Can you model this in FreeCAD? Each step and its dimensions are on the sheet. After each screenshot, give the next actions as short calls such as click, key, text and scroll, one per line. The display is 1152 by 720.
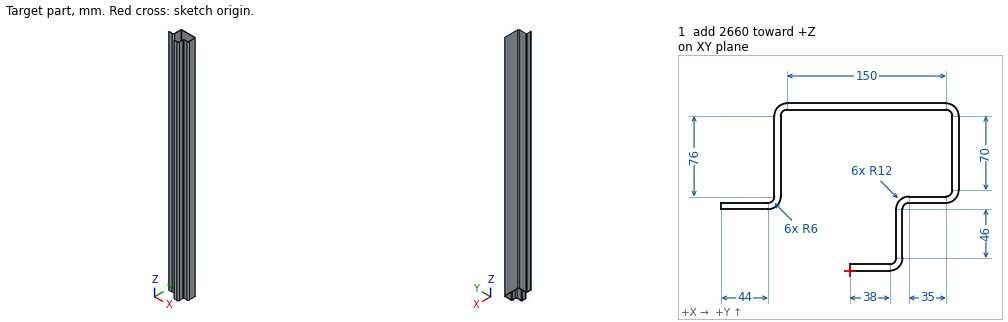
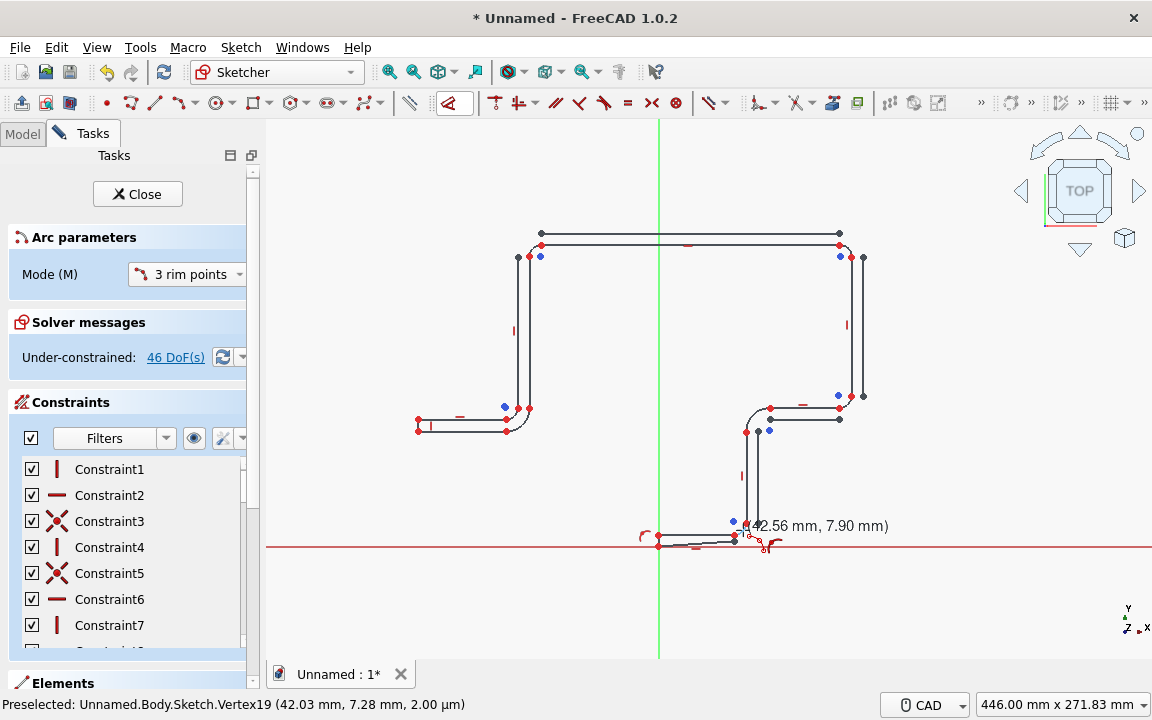
scroll(734, 547, up, 2)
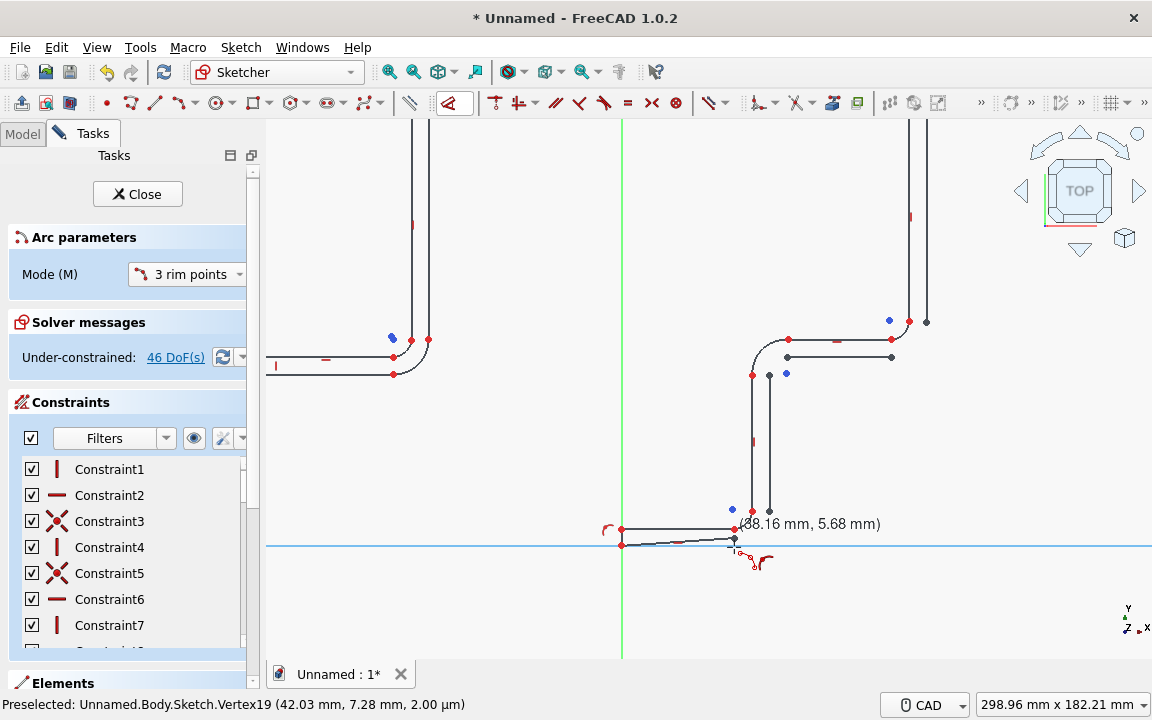
click(735, 538)
click(770, 511)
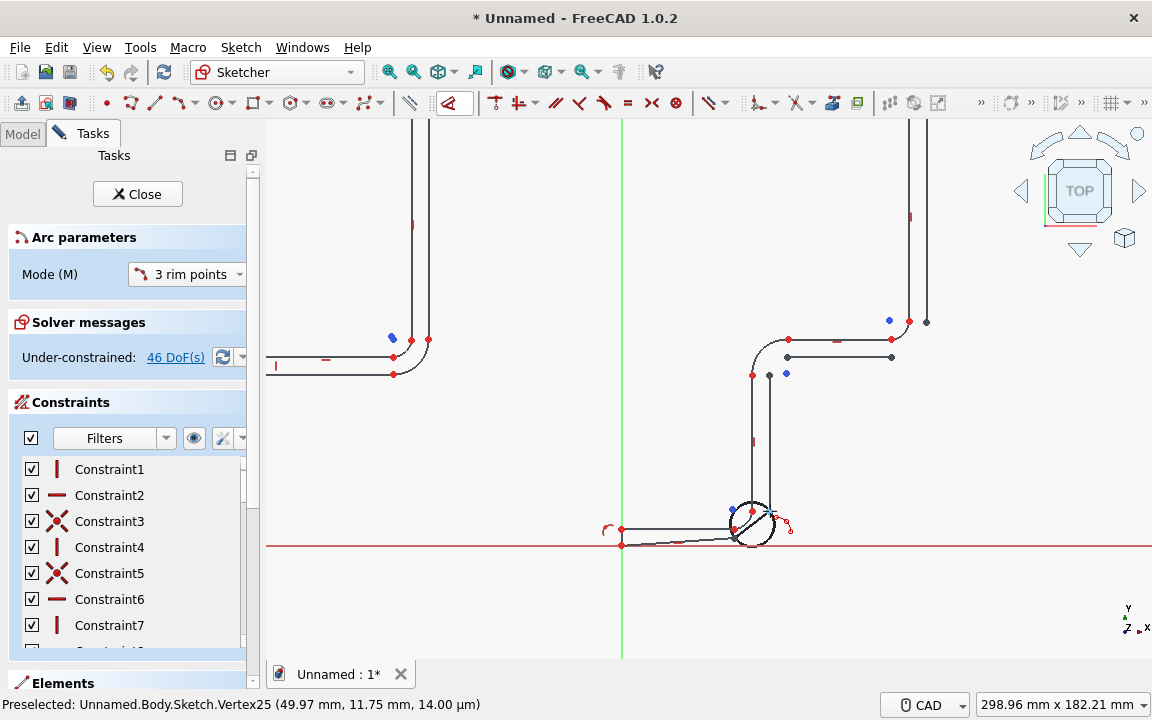
scroll(759, 535, up, 3)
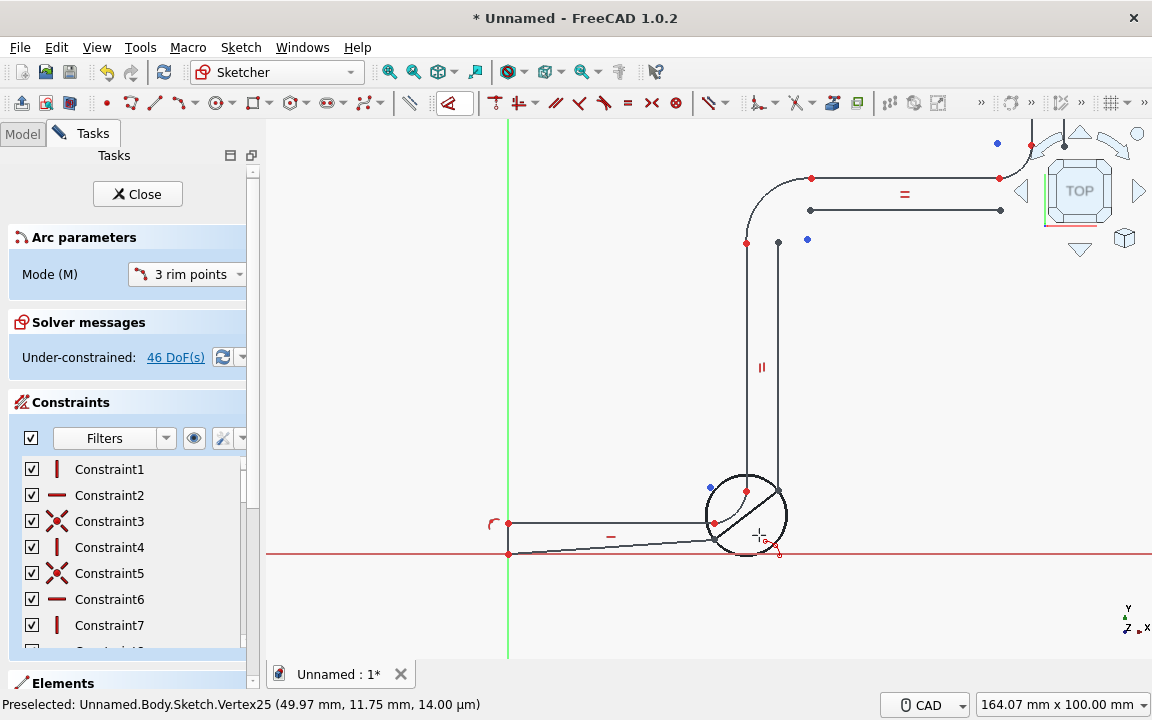
click(759, 535)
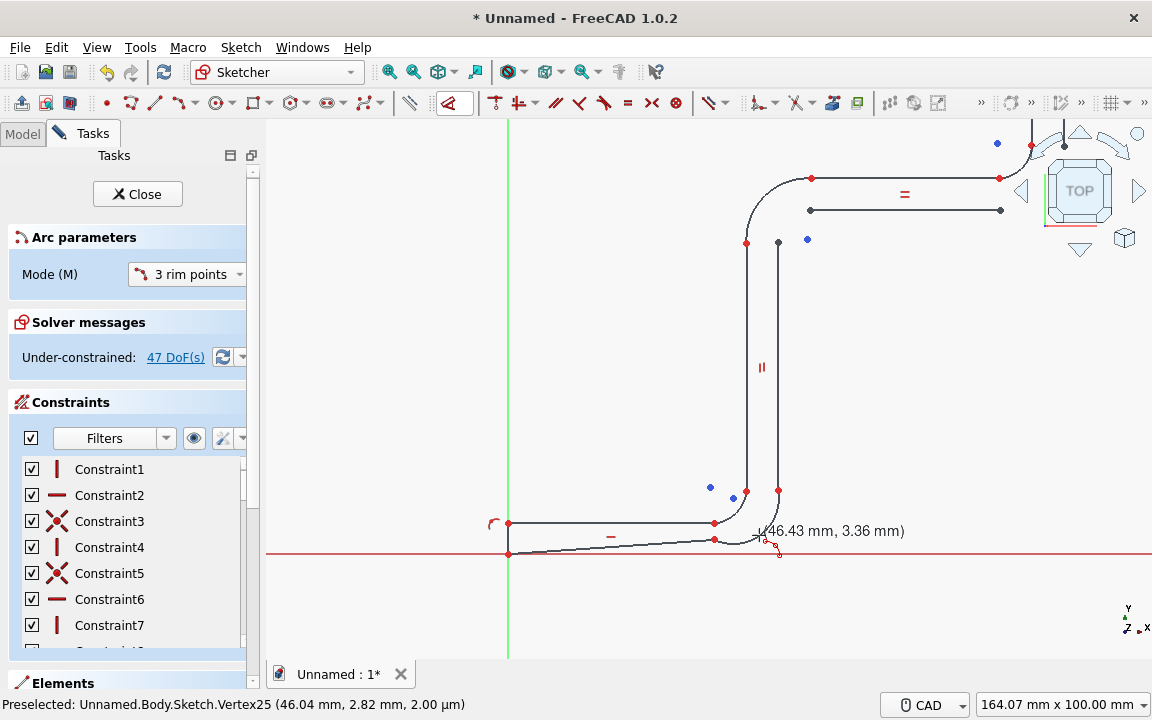
click(778, 243)
click(811, 210)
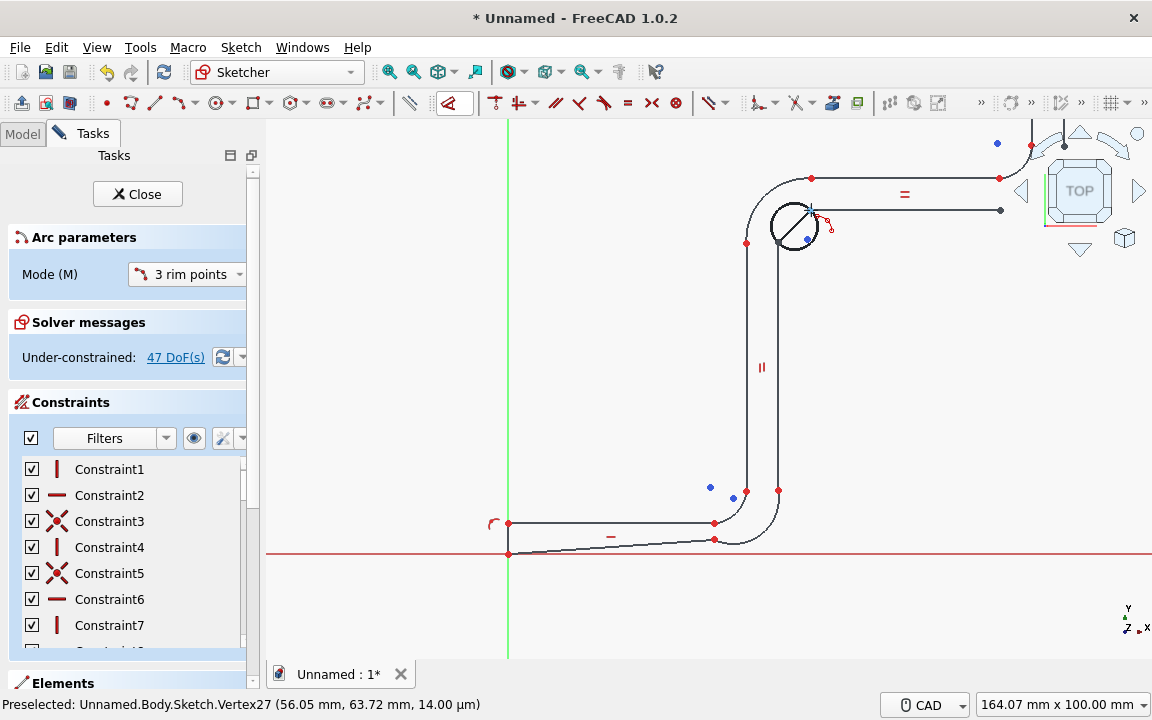
scroll(788, 218, up, 3)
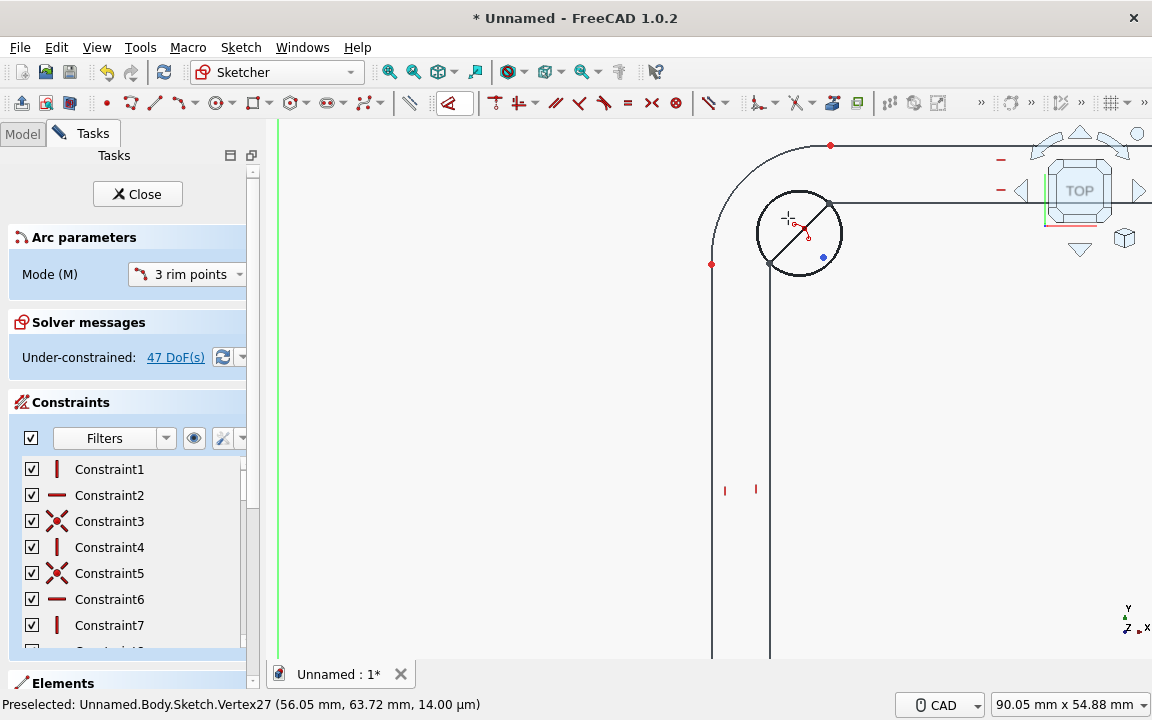
click(787, 218)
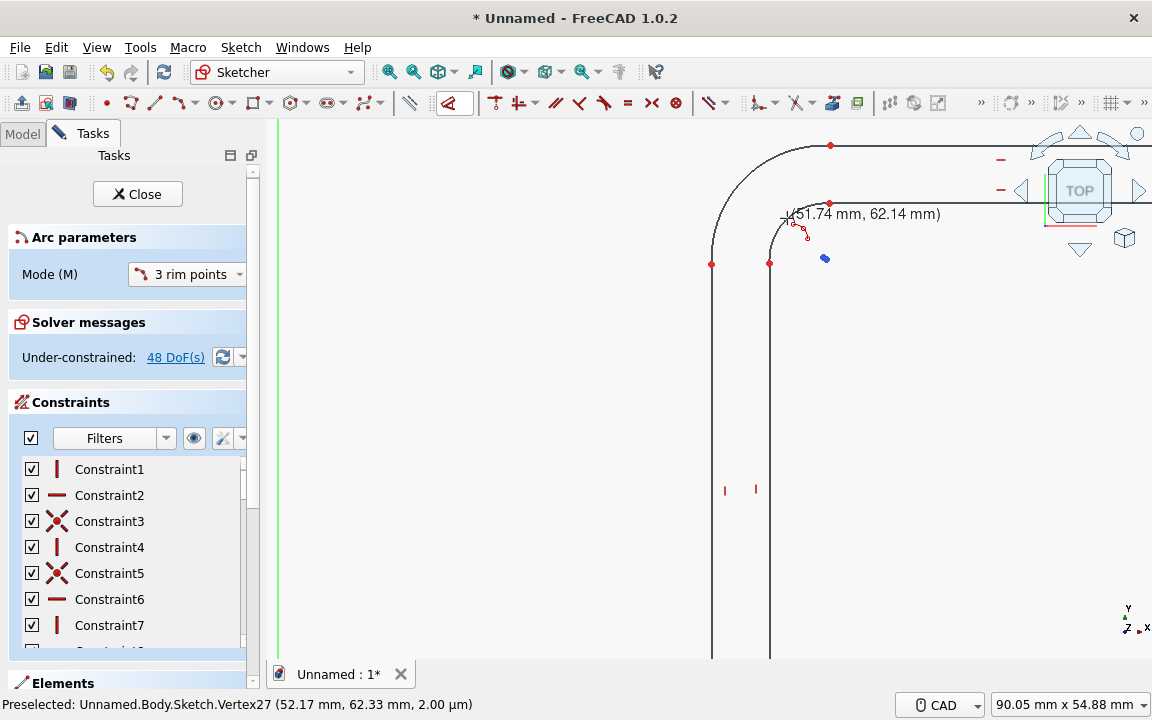
scroll(755, 474, down, 8)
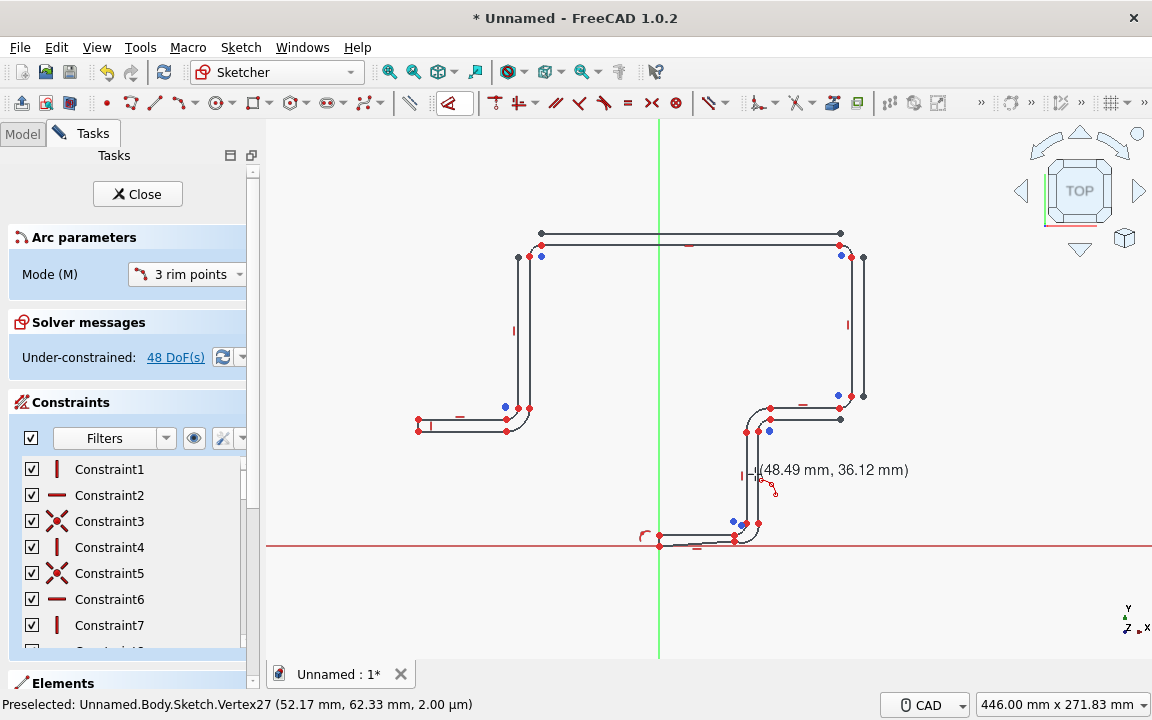
scroll(840, 419, up, 2)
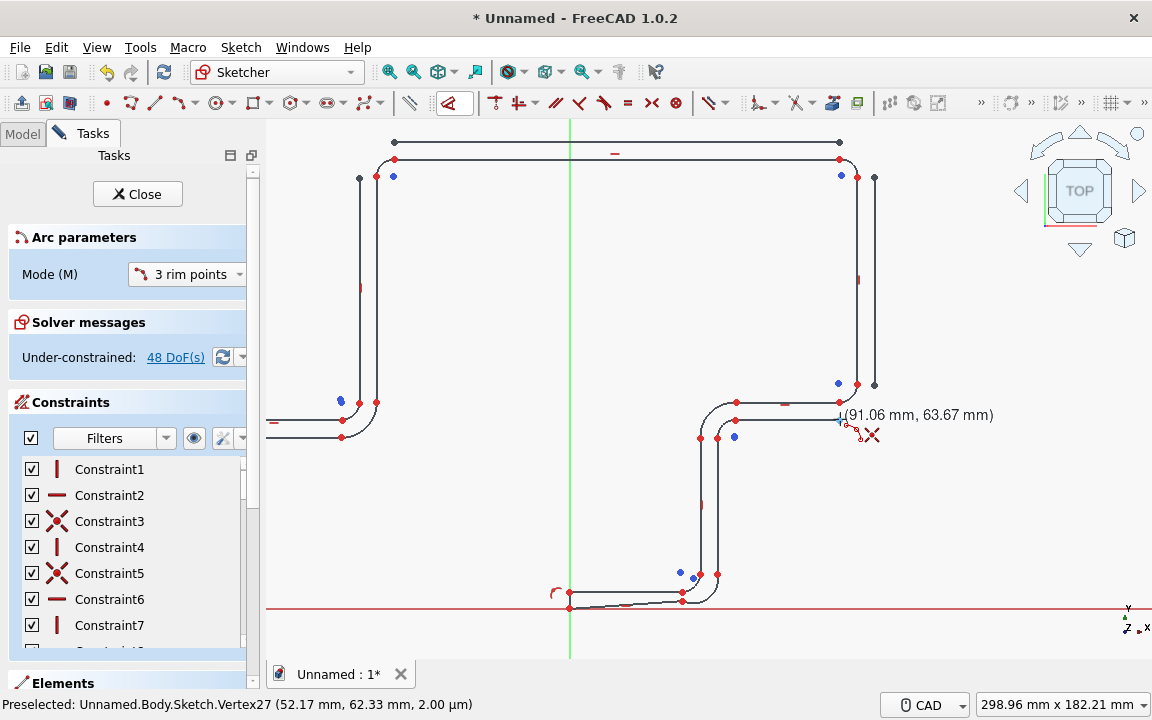
click(840, 420)
click(875, 385)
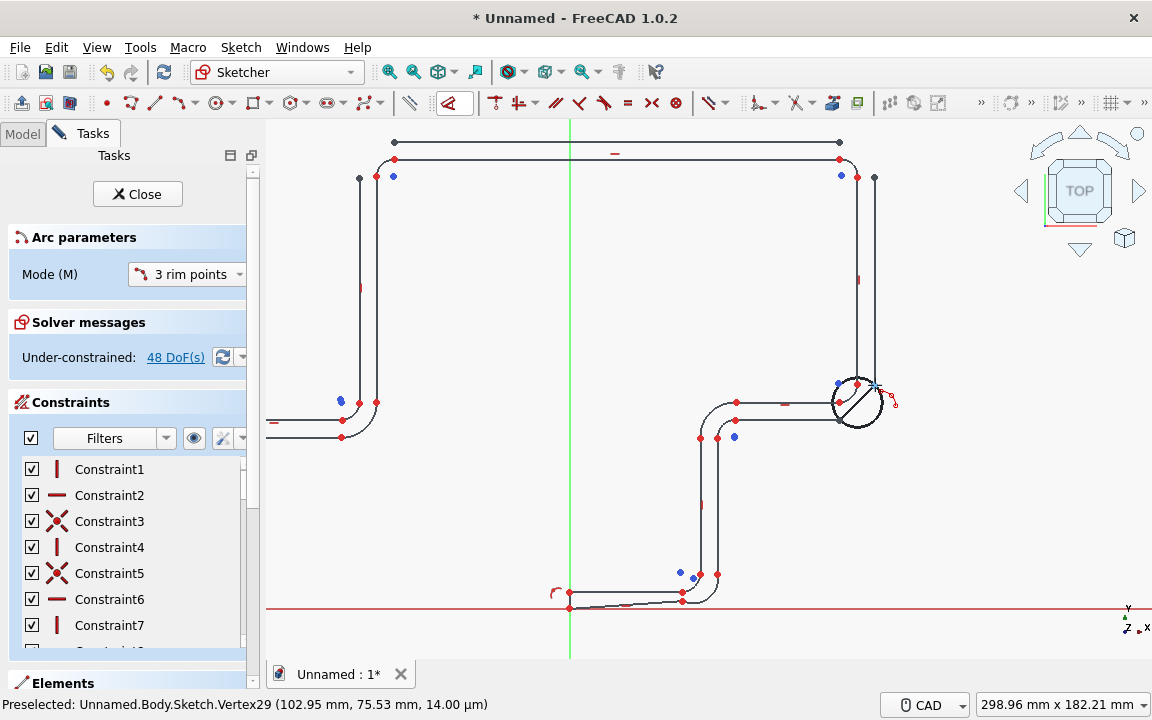
scroll(865, 409, up, 3)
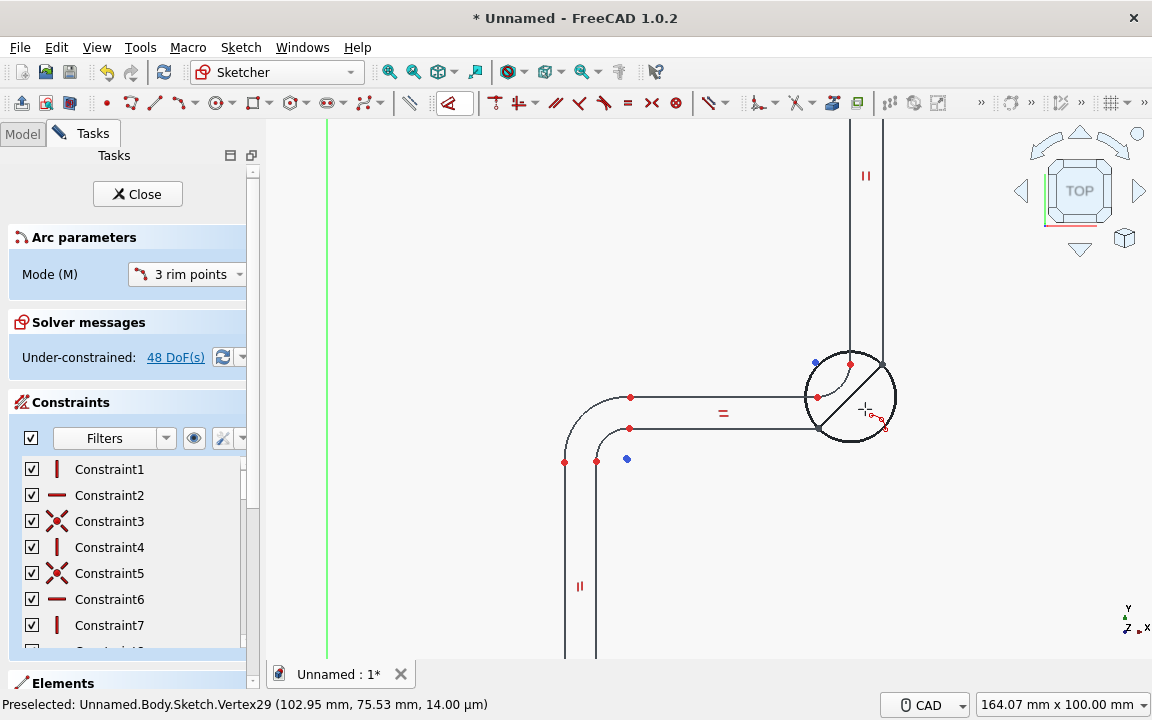
click(864, 408)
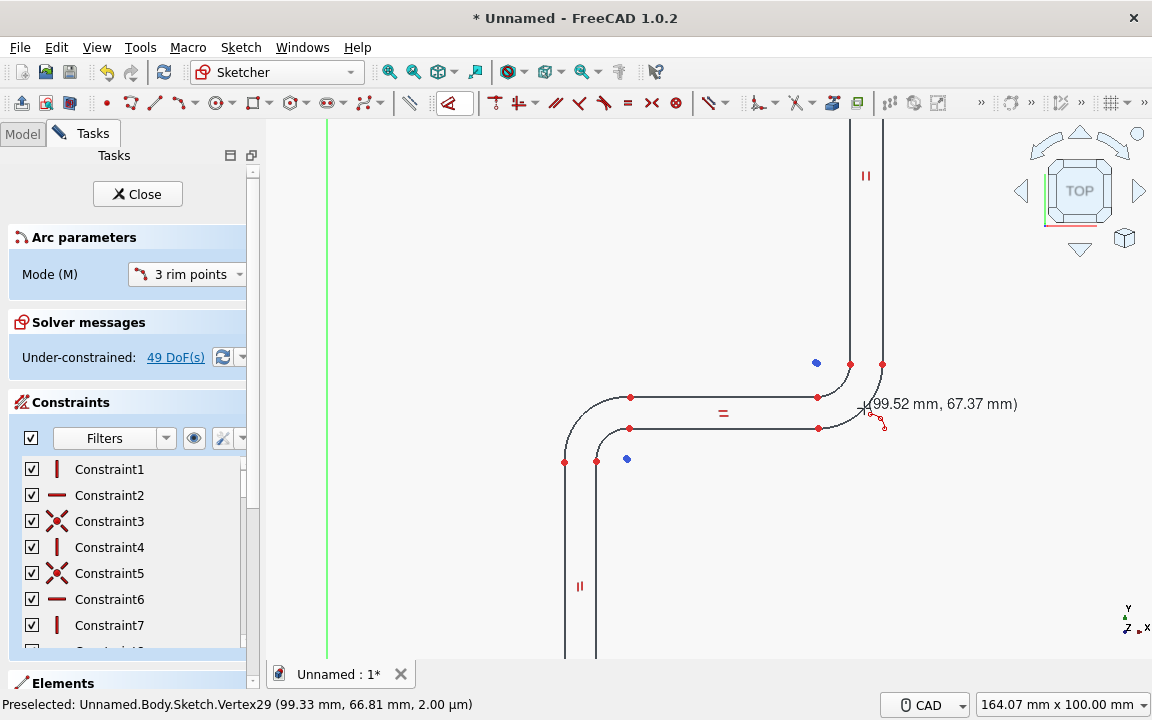
scroll(851, 414, down, 5)